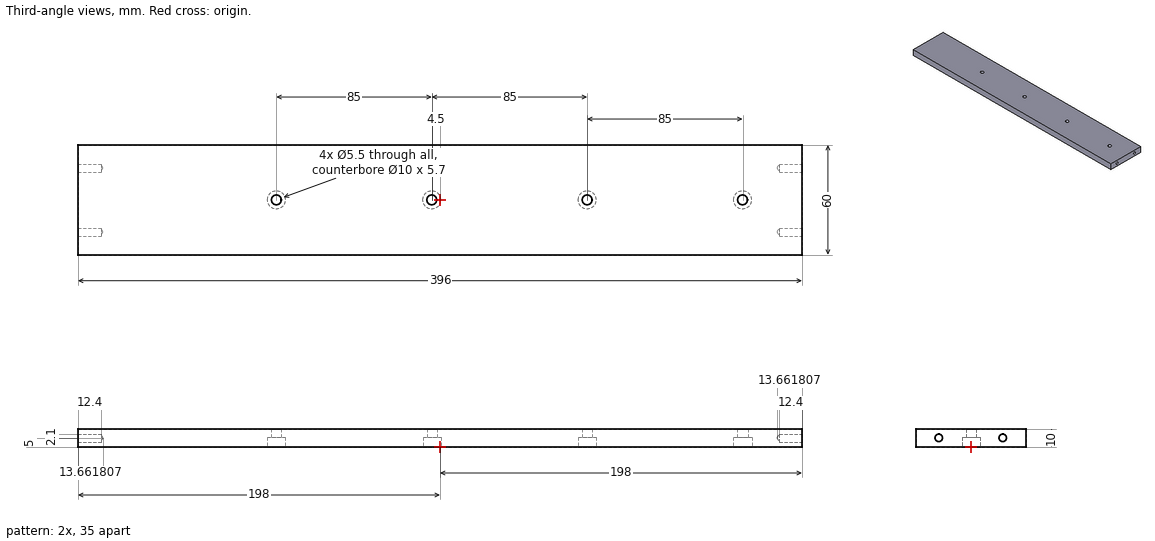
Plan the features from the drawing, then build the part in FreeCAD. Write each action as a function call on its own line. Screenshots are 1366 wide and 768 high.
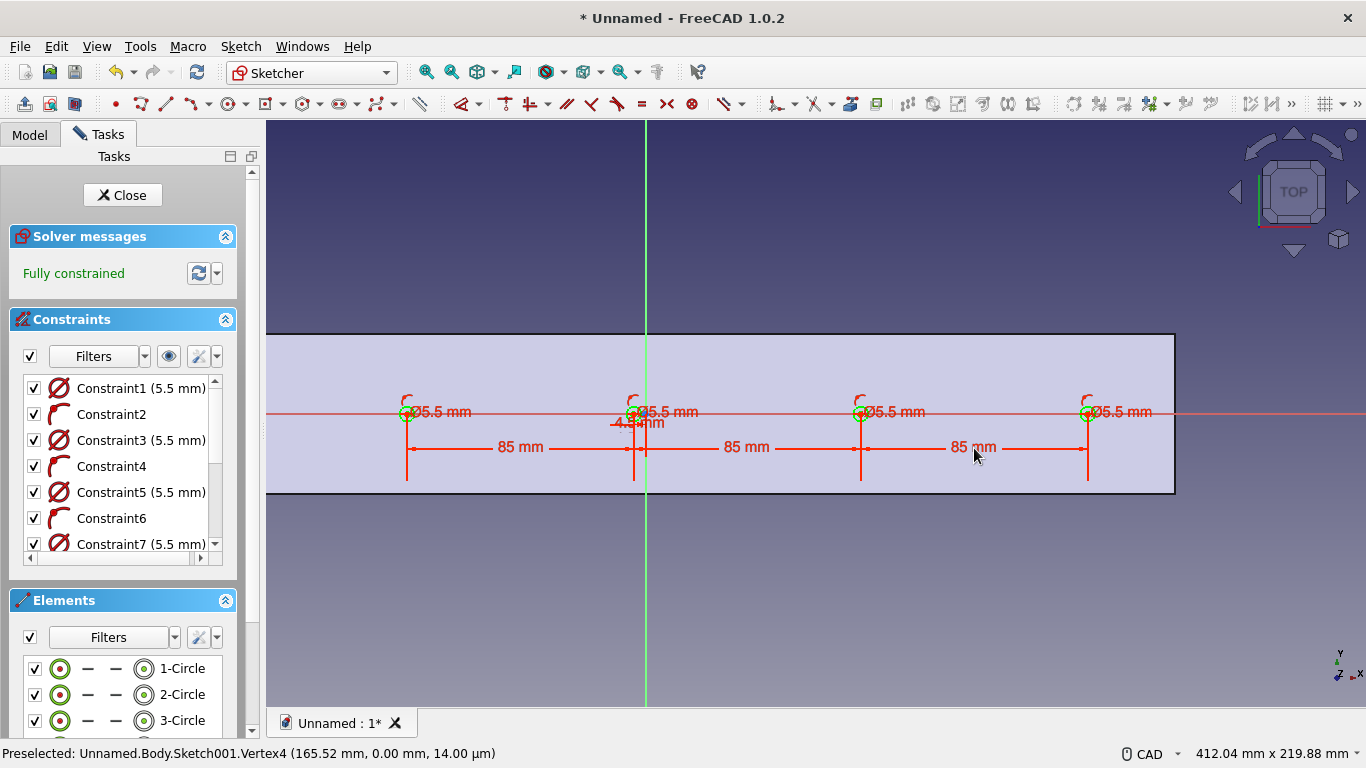
click(123, 195)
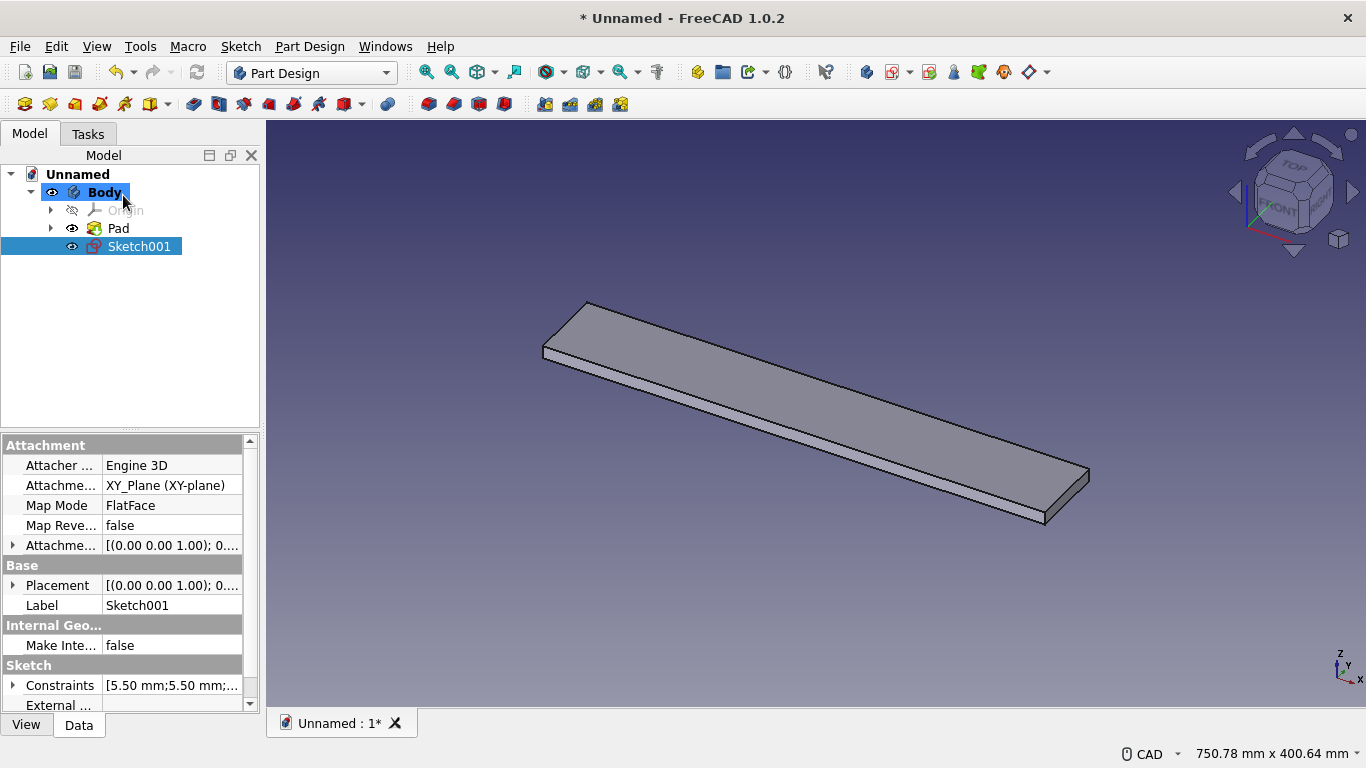
click(219, 104)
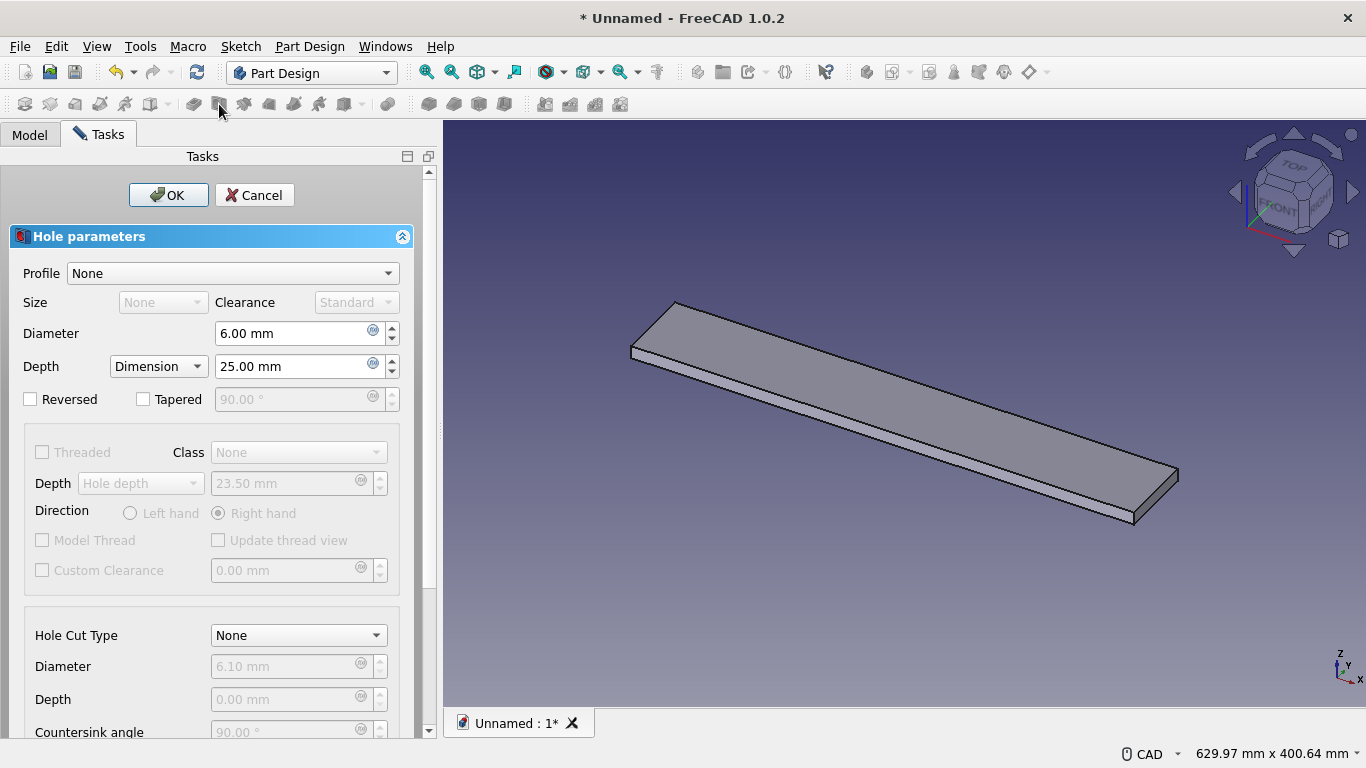
triple_click(300, 334)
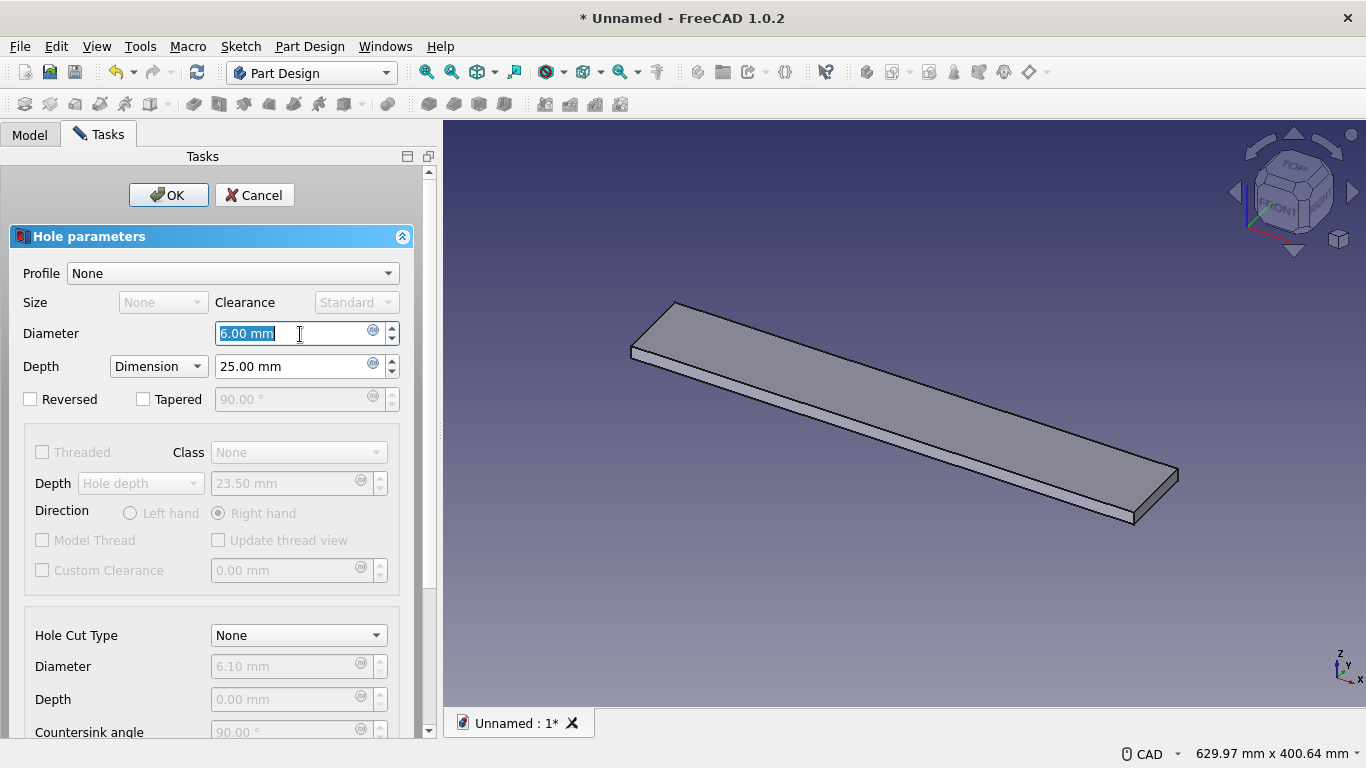
text(5.5)
key(Tab)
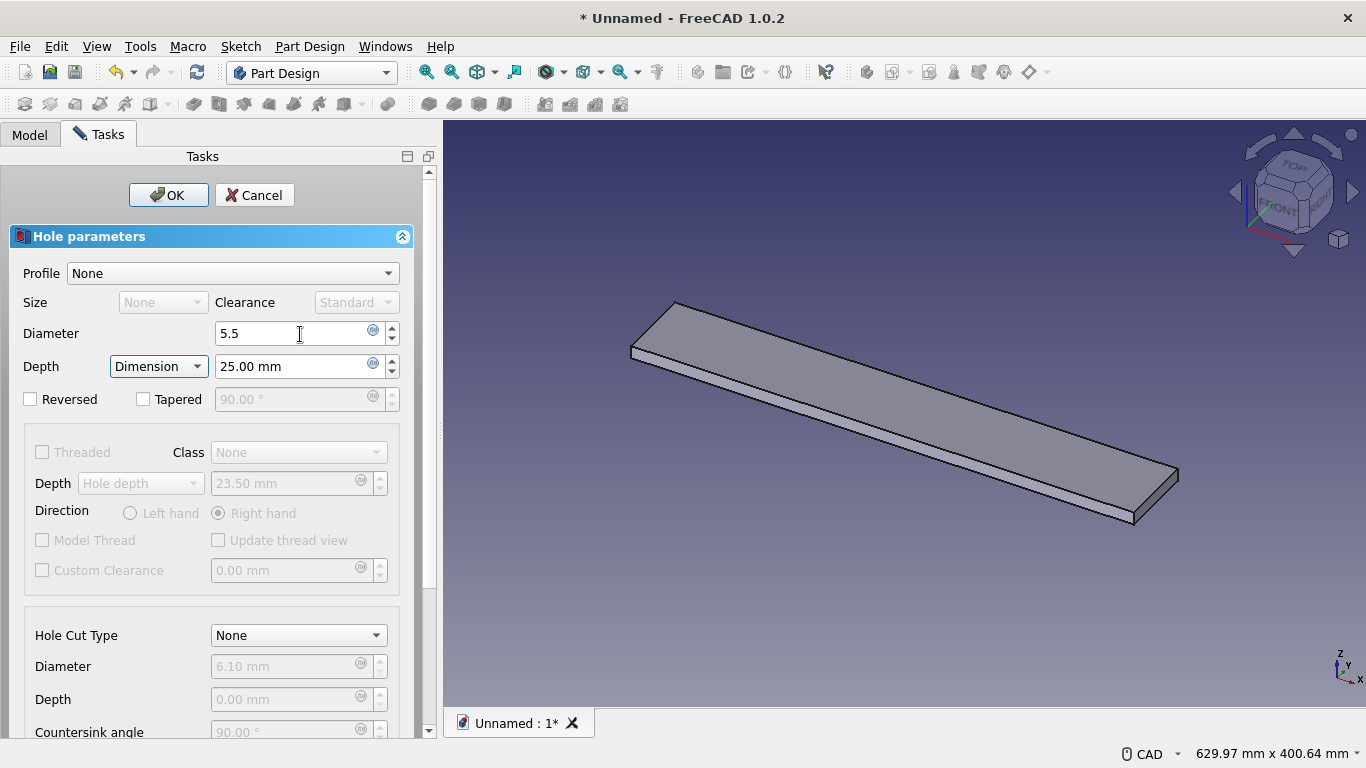
click(160, 366)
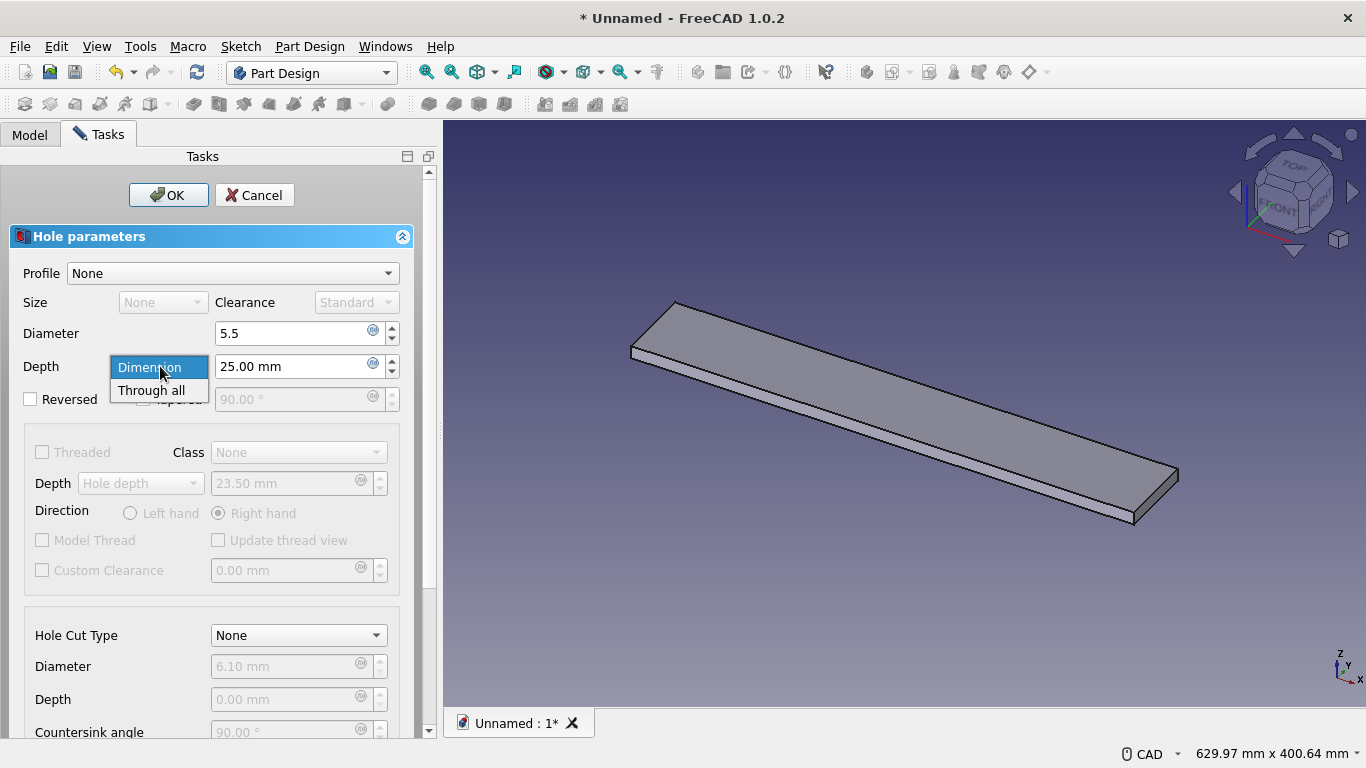
click(158, 390)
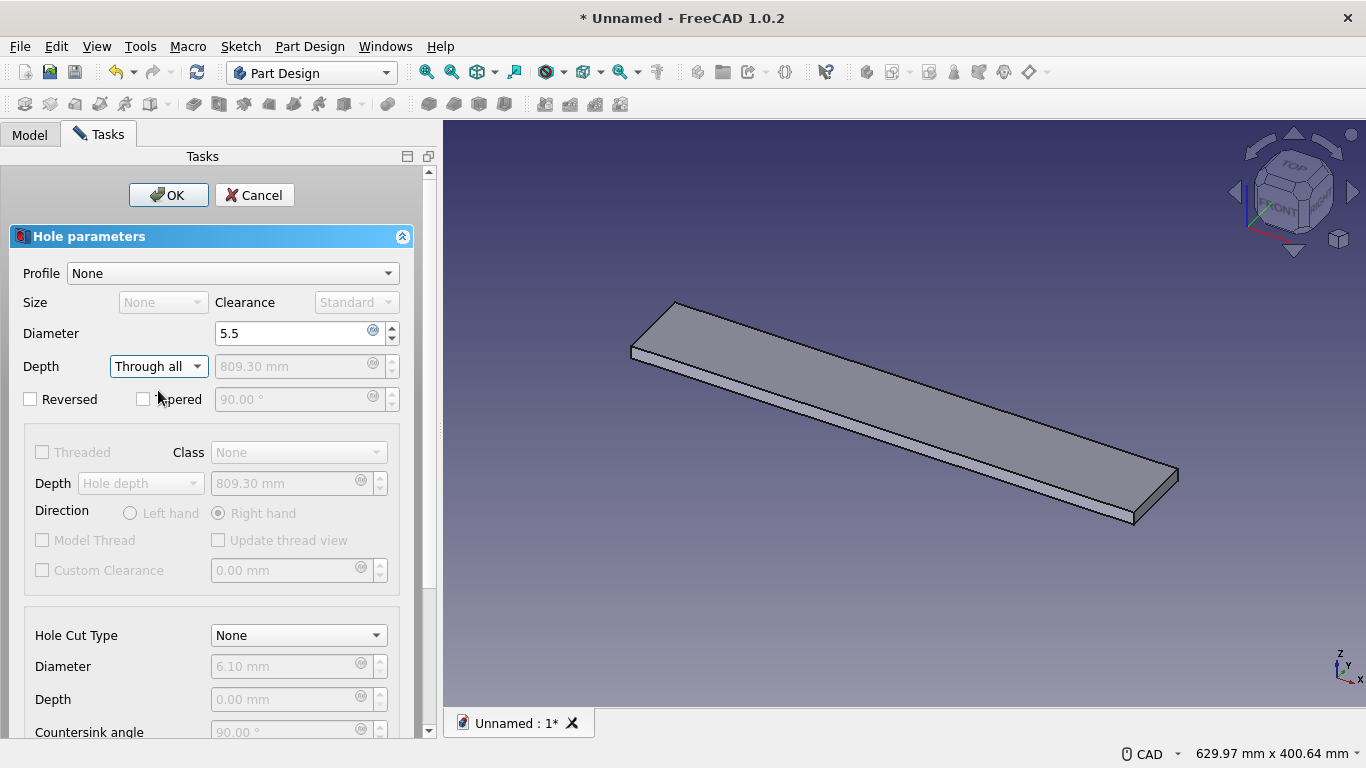
click(31, 399)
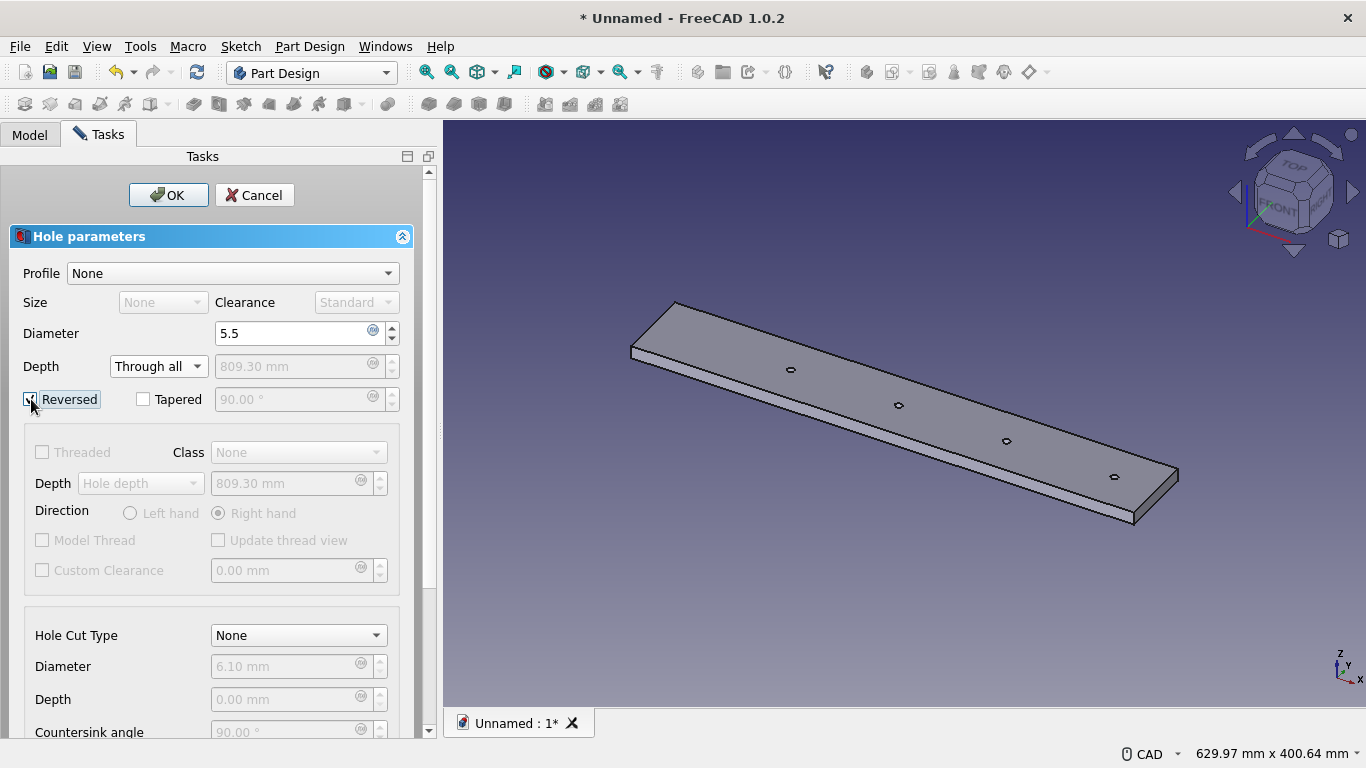
click(300, 636)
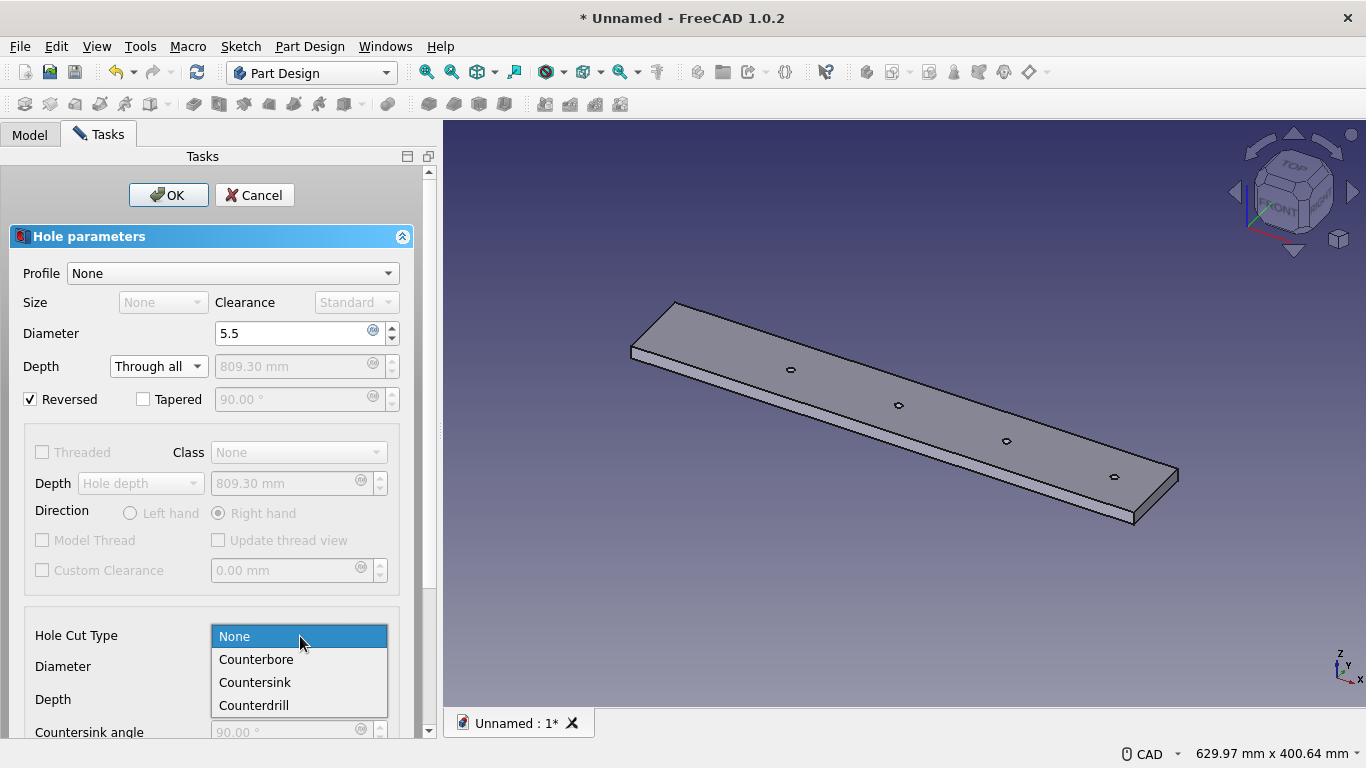
click(298, 660)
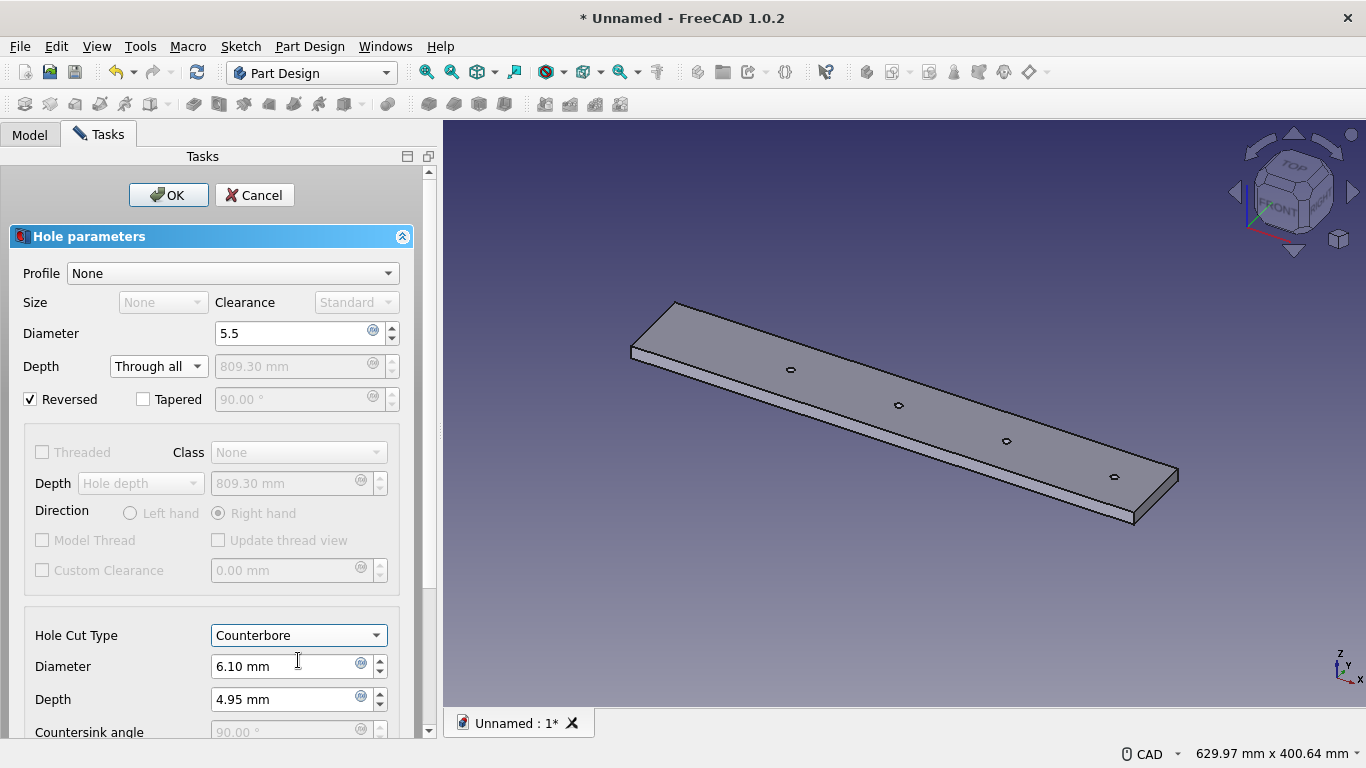
triple_click(292, 666)